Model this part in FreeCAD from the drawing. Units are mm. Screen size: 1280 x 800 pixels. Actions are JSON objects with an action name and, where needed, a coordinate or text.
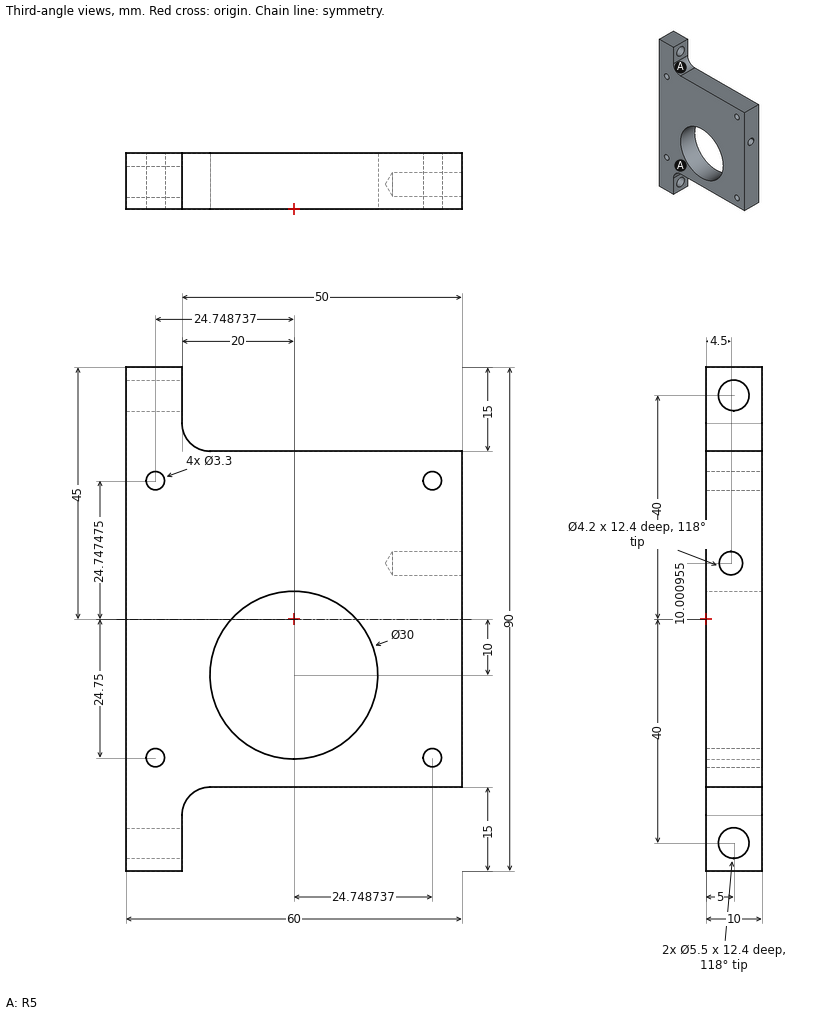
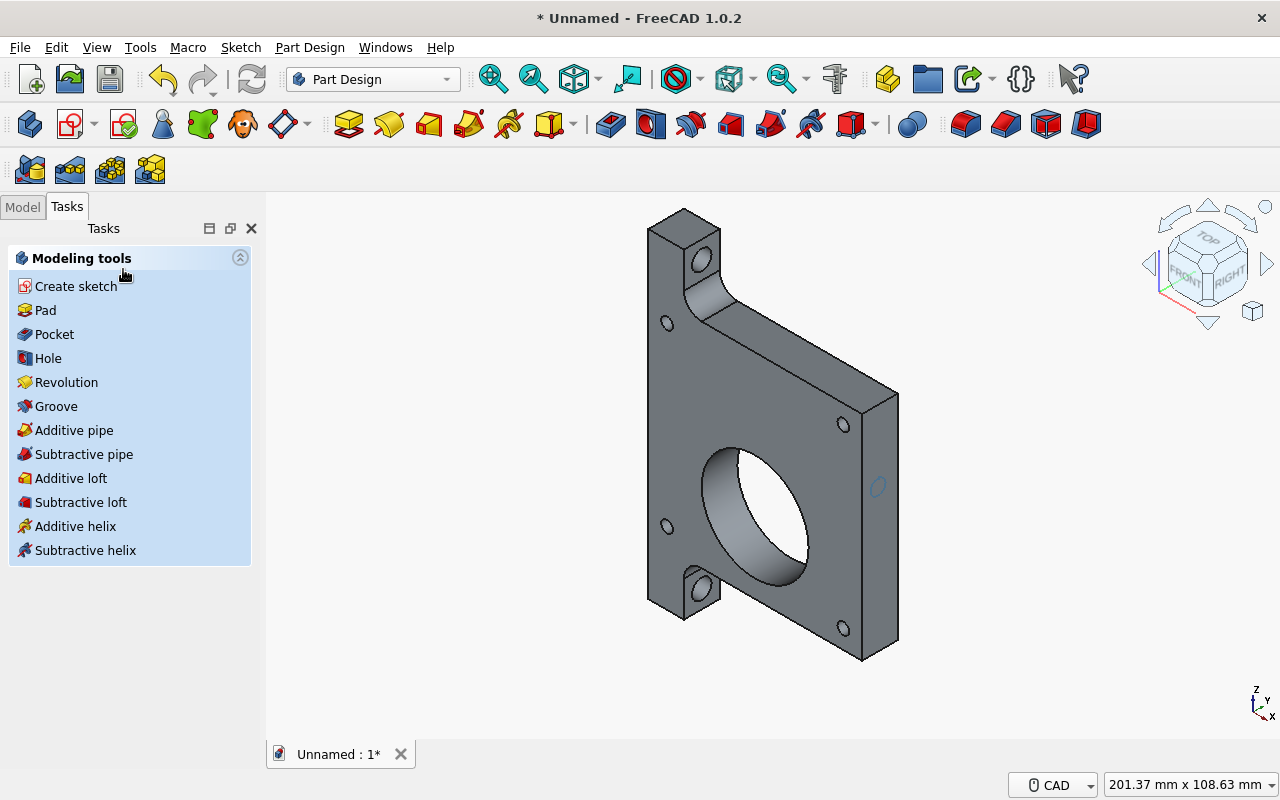
{"action": "left_click", "coordinate": [652, 124]}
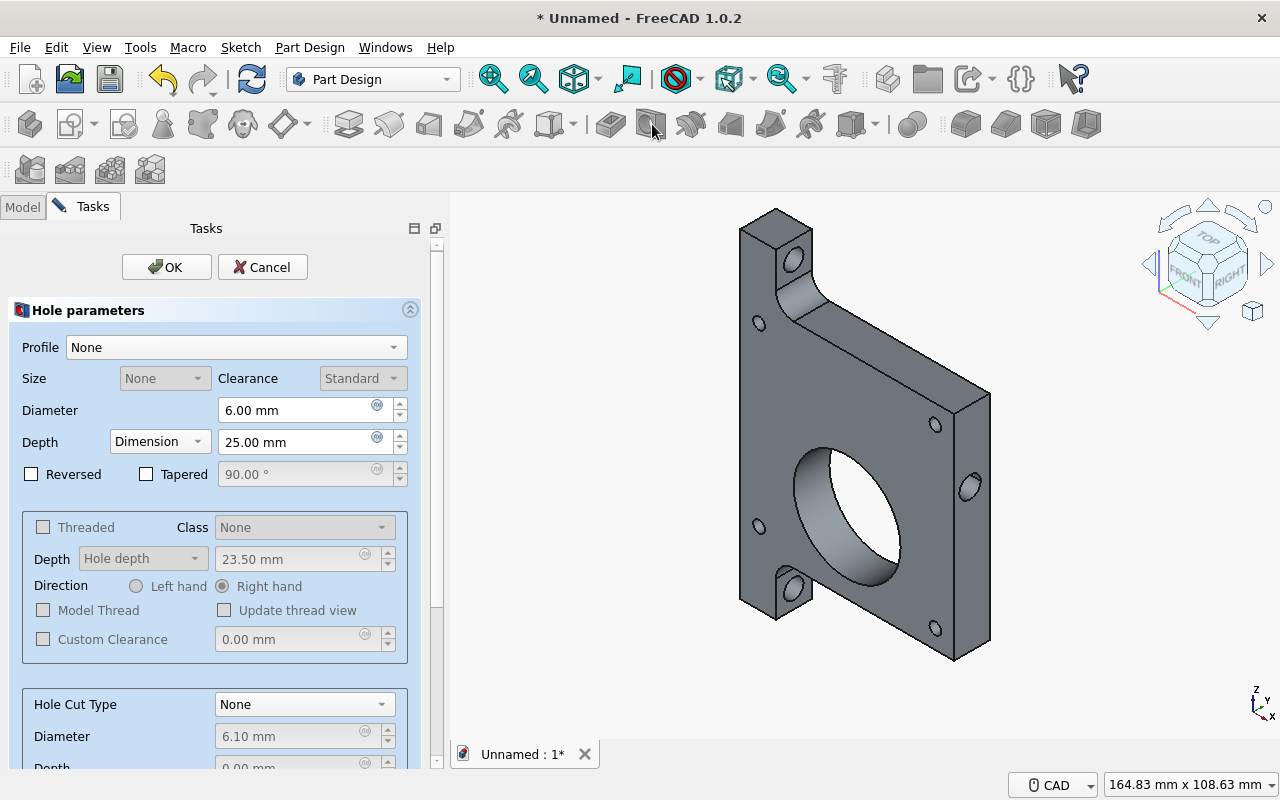
{"action": "triple_click", "coordinate": [305, 410]}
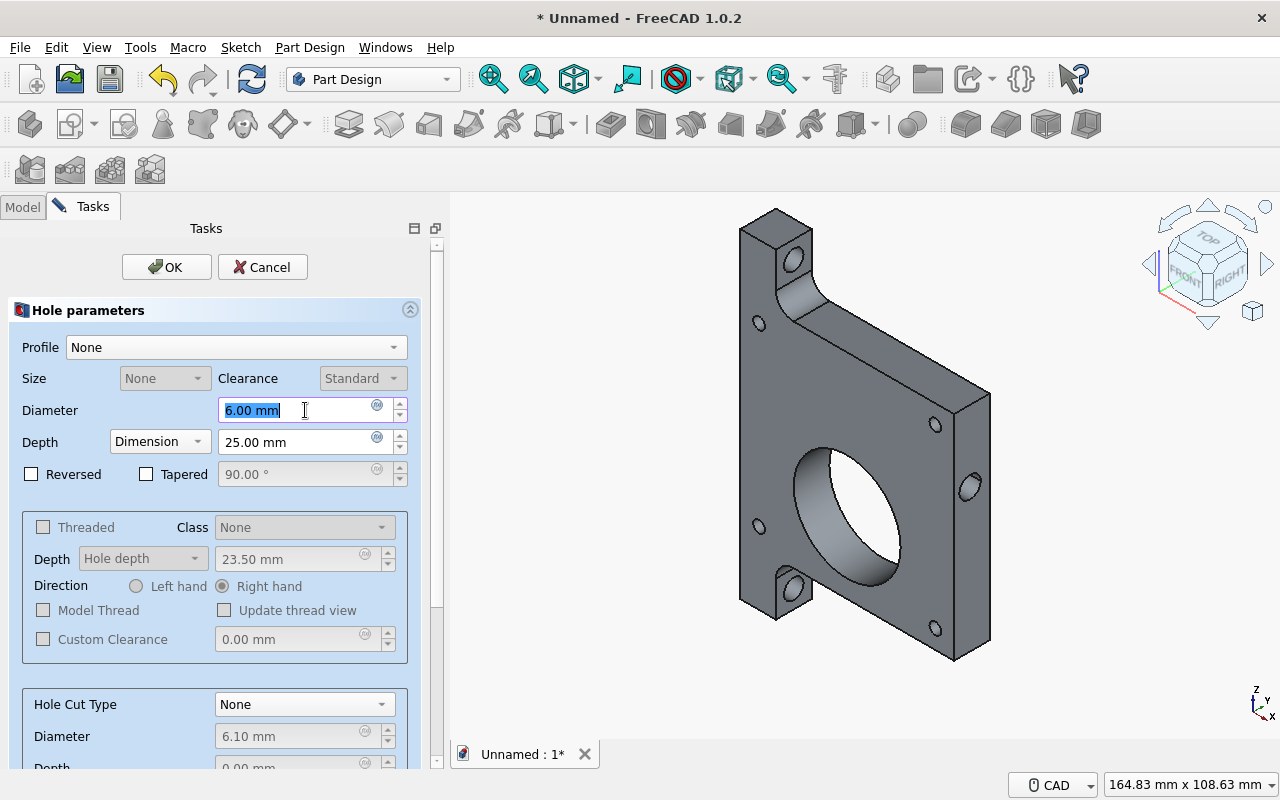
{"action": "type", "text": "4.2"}
{"action": "key", "text": "Tab"}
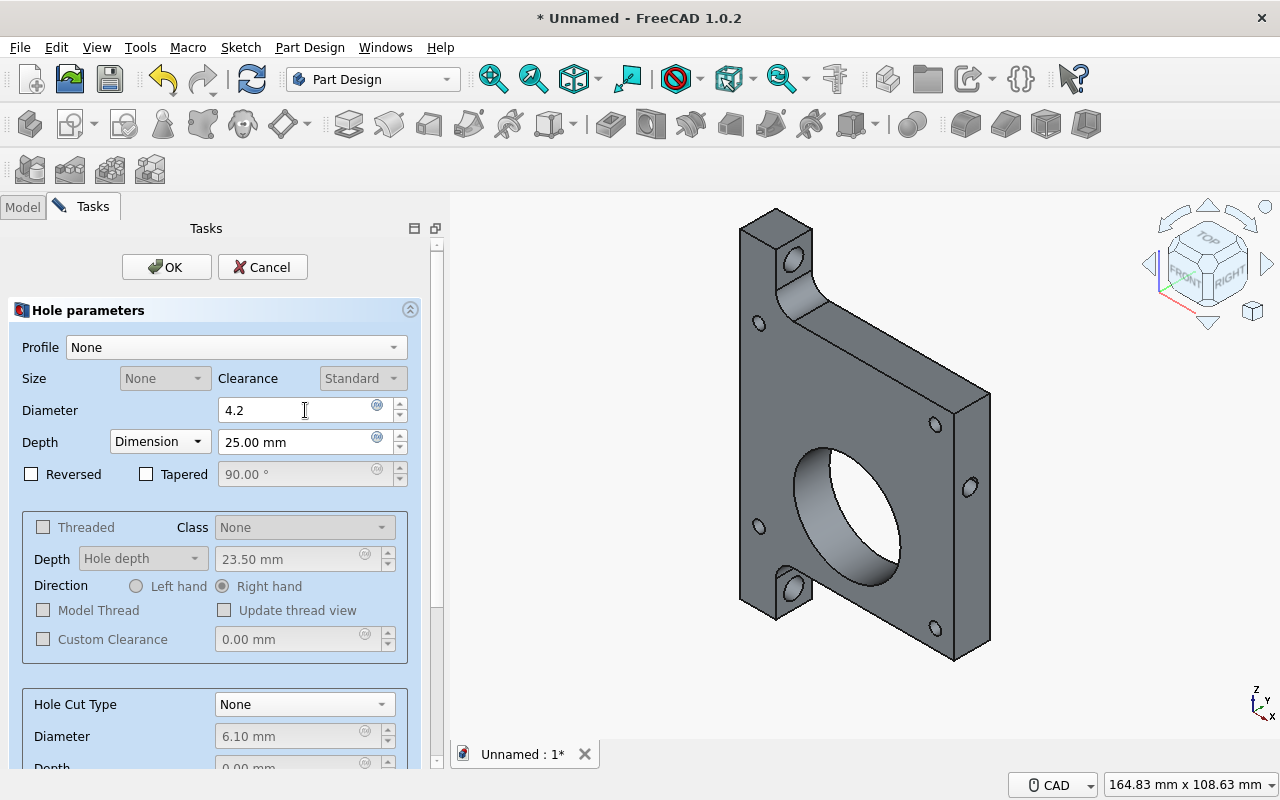
{"action": "triple_click", "coordinate": [305, 442]}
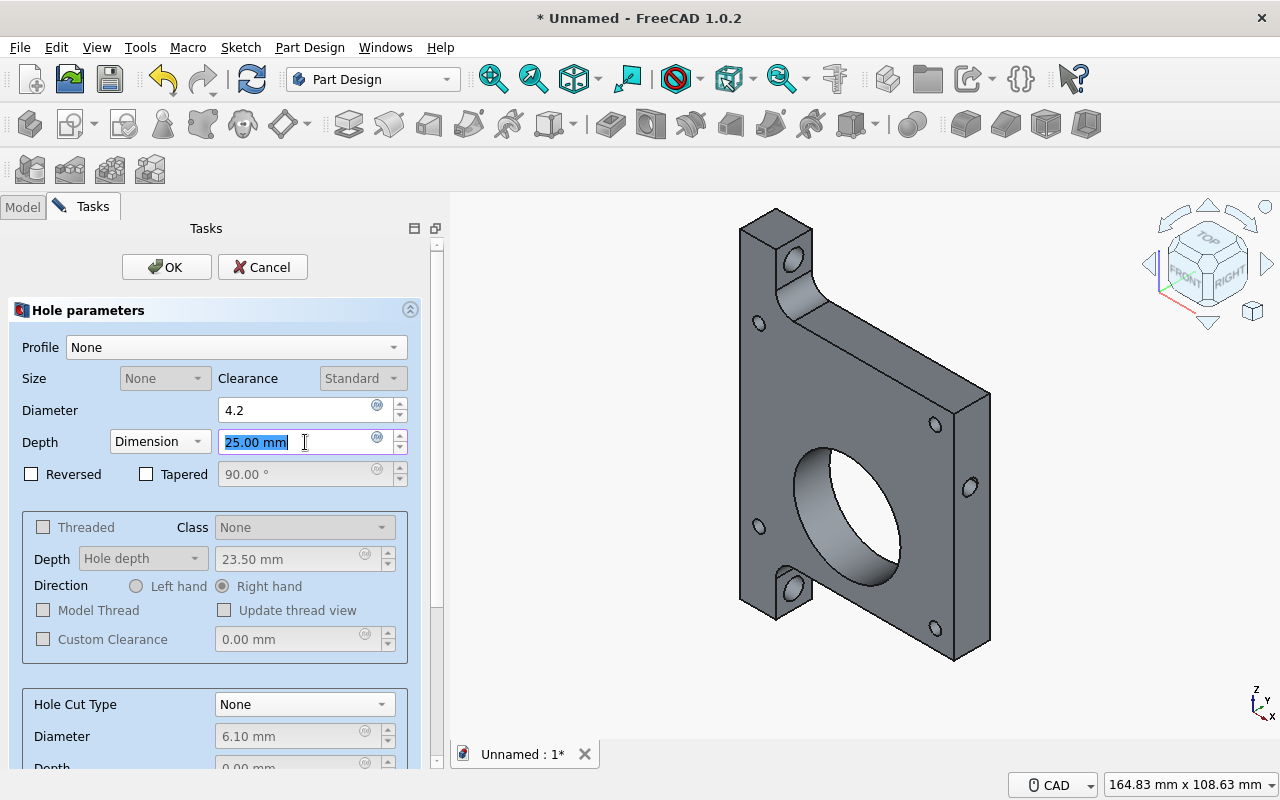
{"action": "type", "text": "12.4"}
{"action": "key", "text": "Tab"}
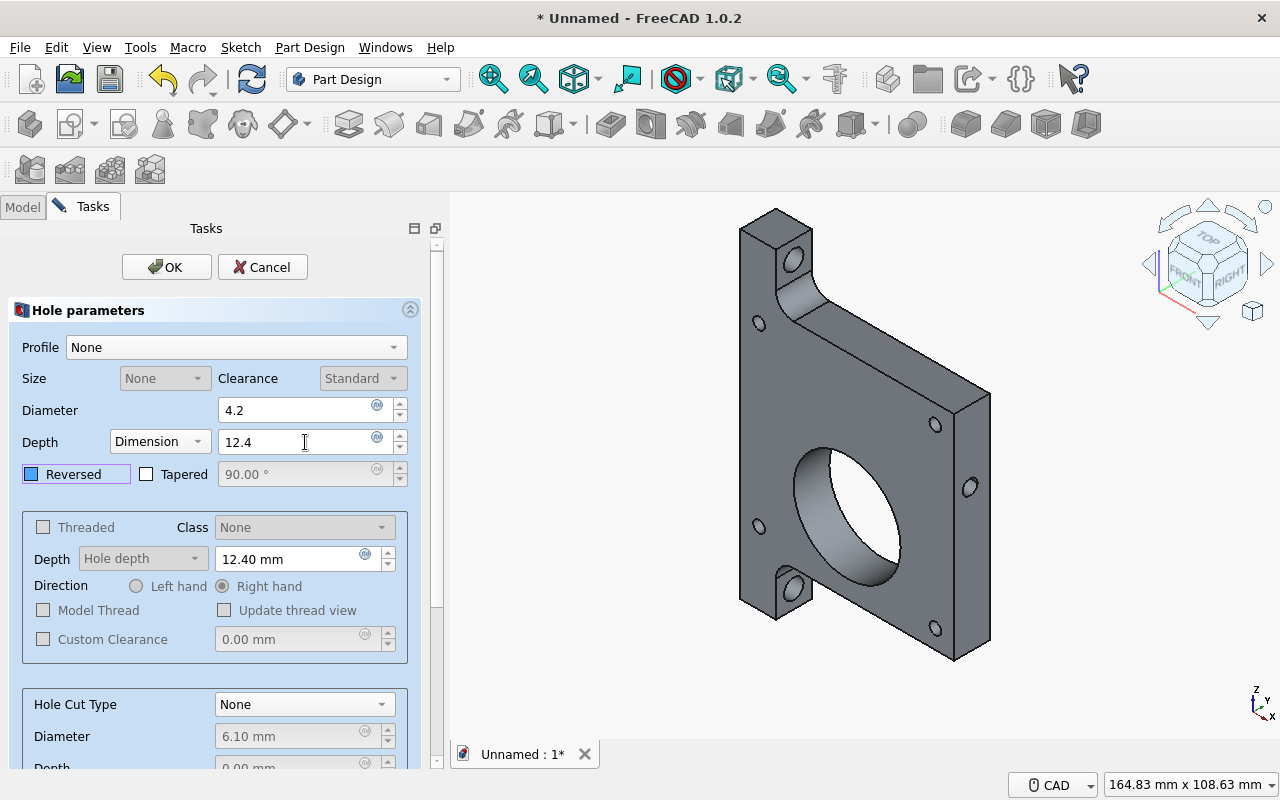
{"action": "left_click", "coordinate": [167, 267]}